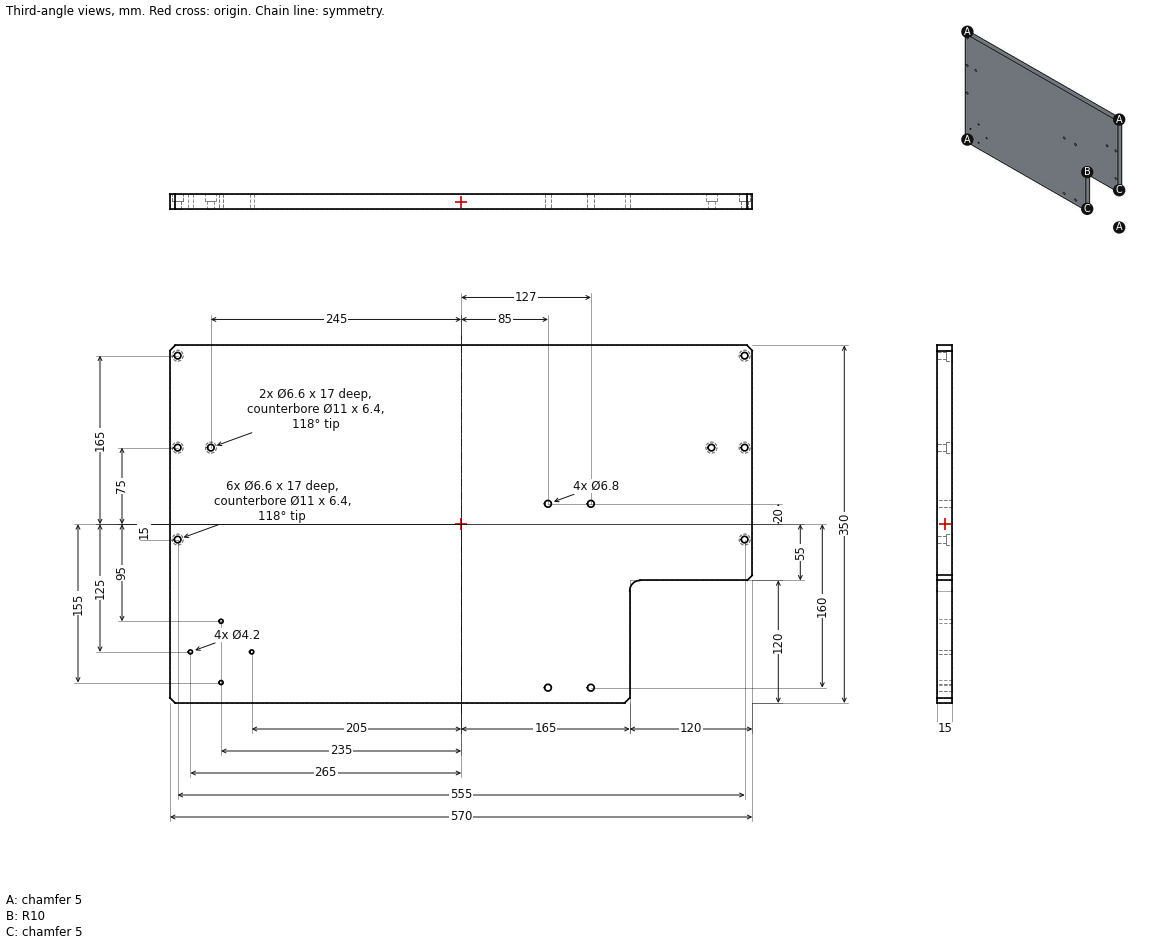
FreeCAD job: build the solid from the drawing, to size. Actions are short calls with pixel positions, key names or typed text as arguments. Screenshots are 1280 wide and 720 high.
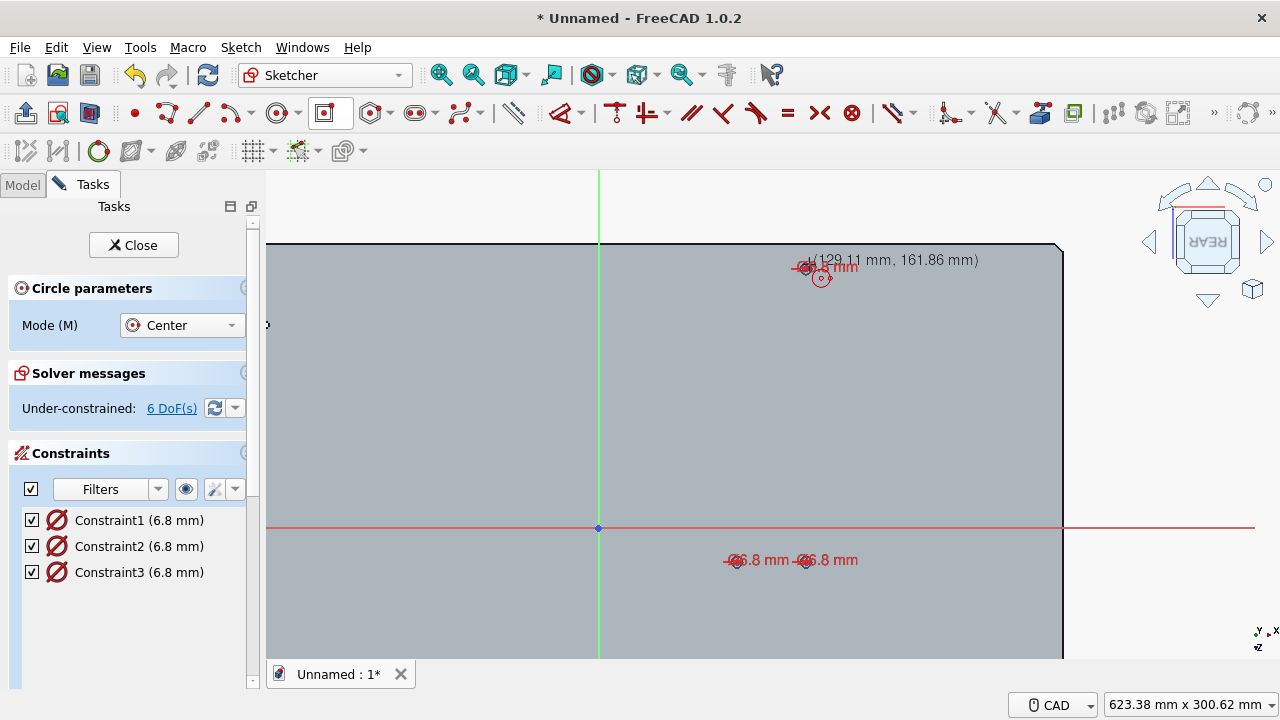
scroll(737, 268, up, 8)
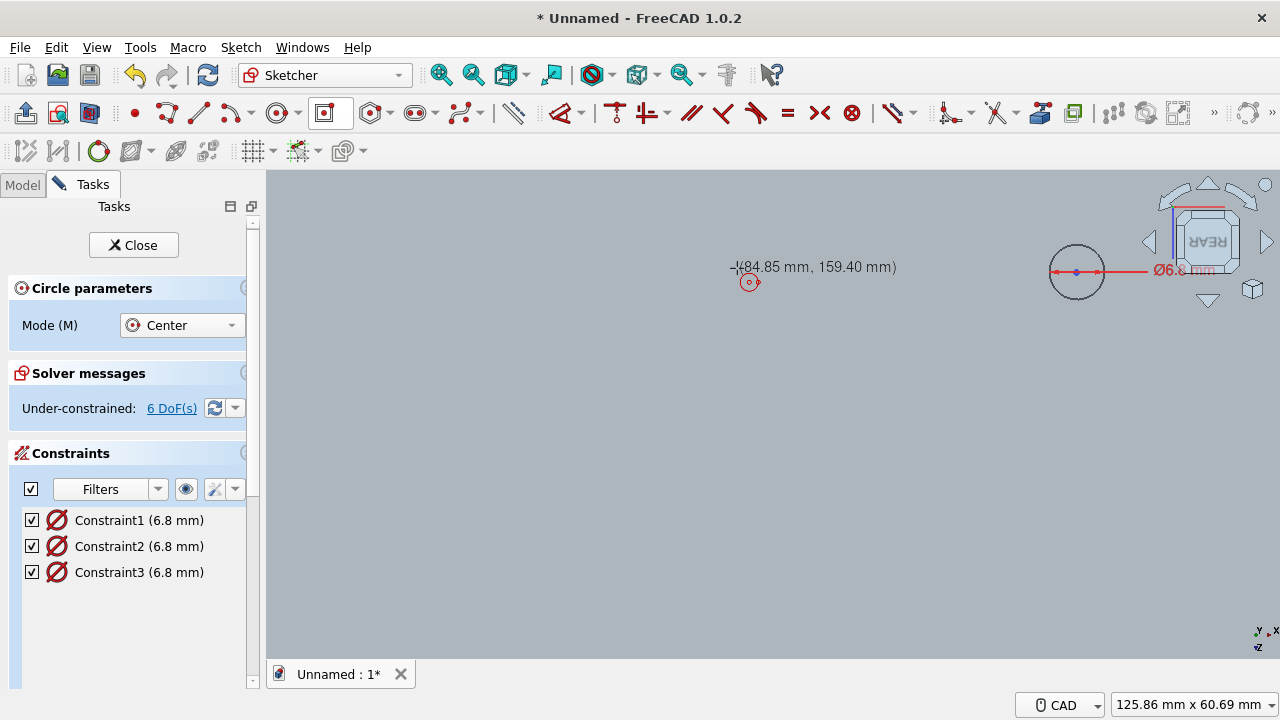
scroll(737, 268, down, 8)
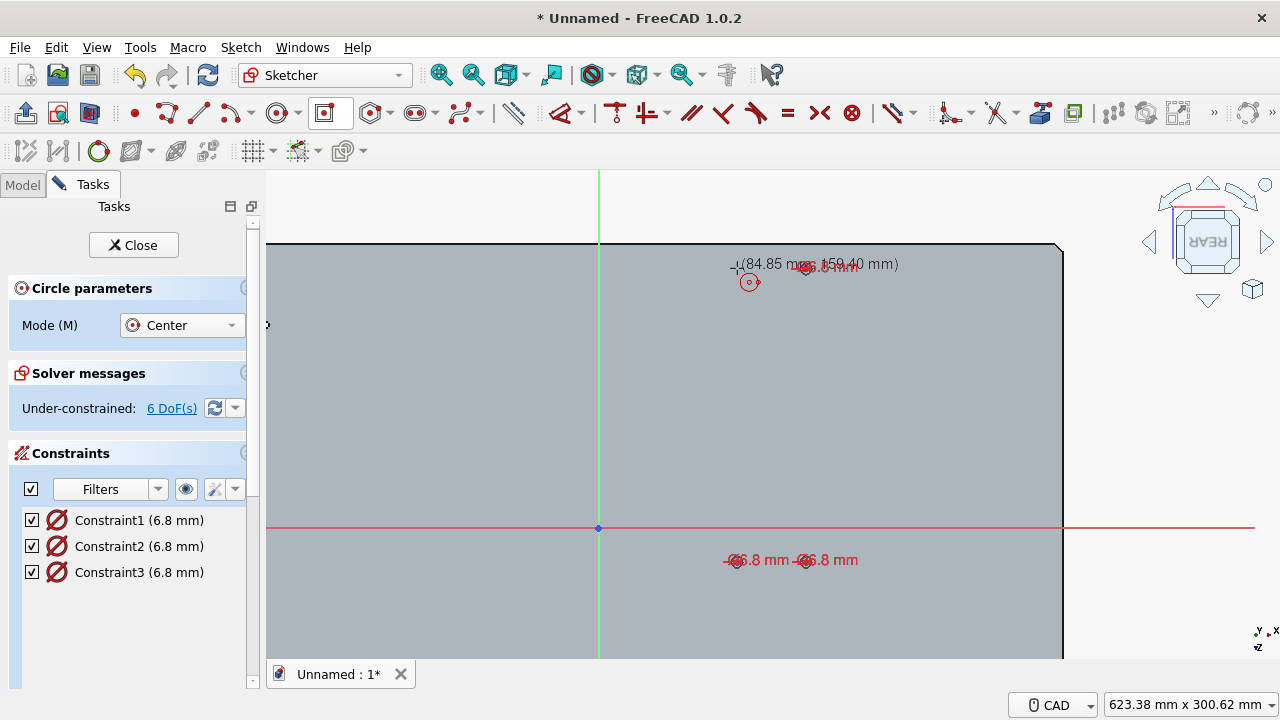
click(737, 268)
move(741, 264)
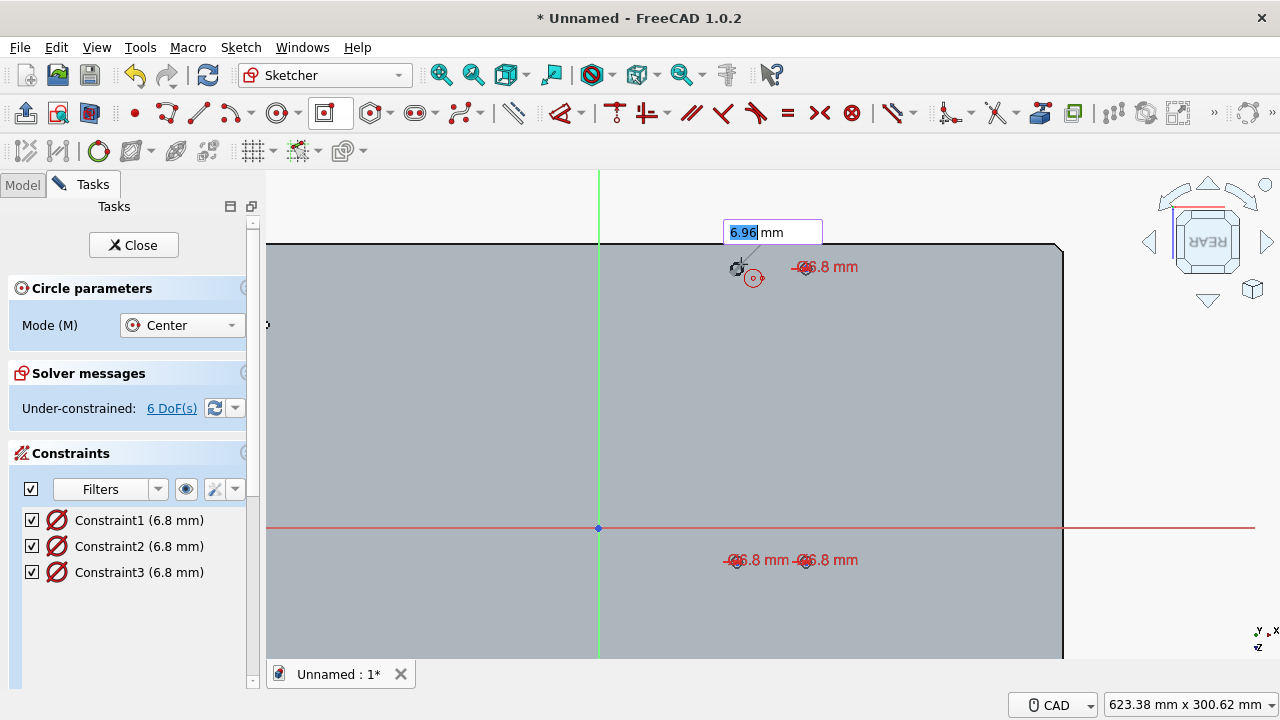
text(6.8)
key(Return)
key(Escape)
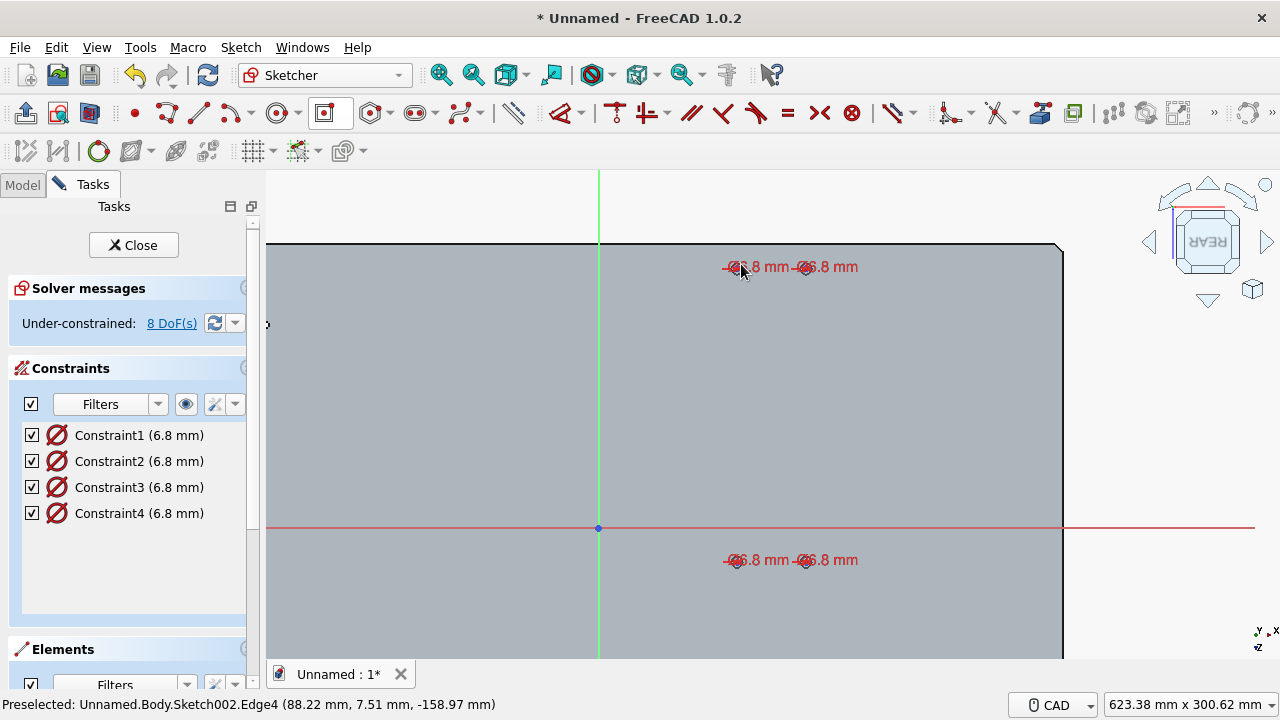
click(560, 114)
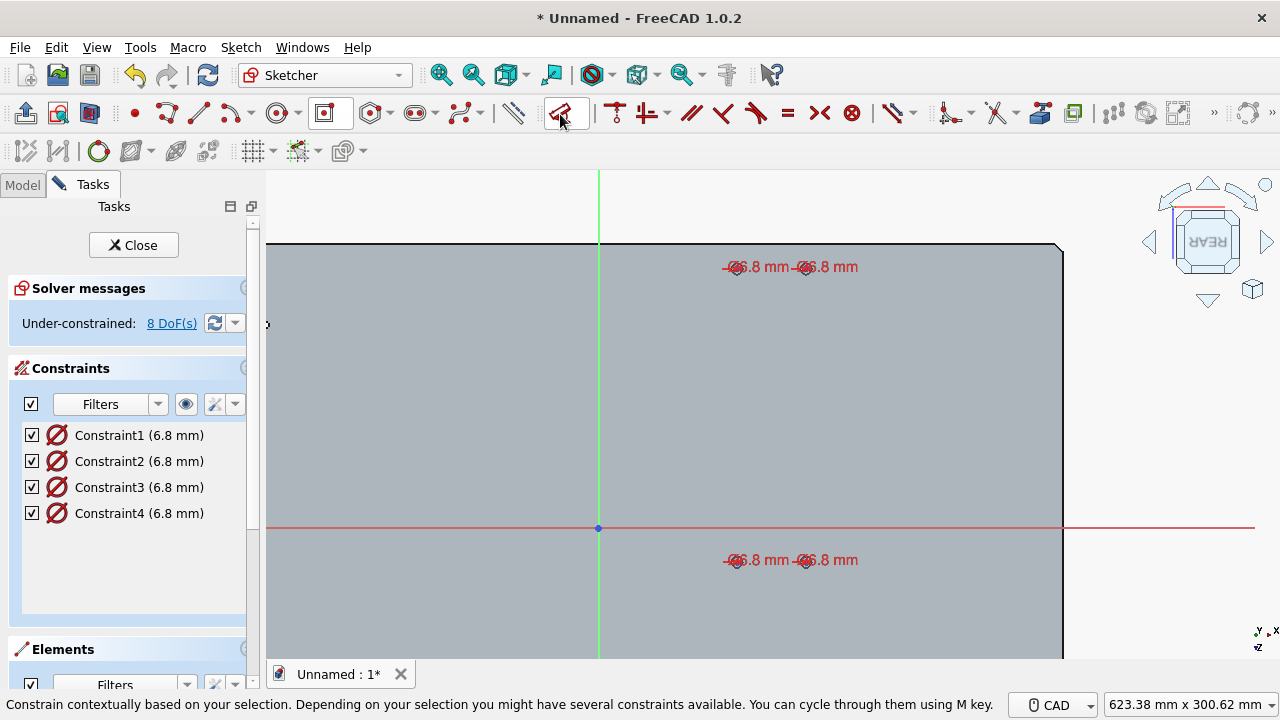
click(737, 562)
click(668, 596)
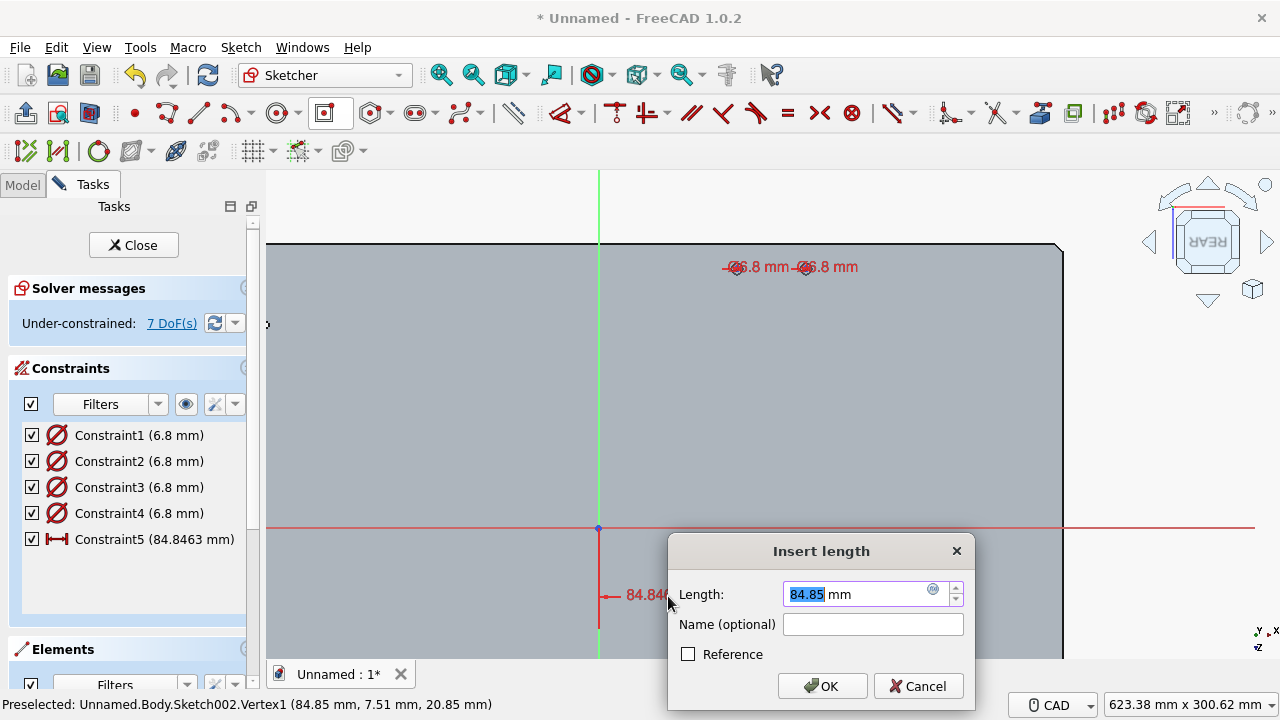
text(85)
key(Return)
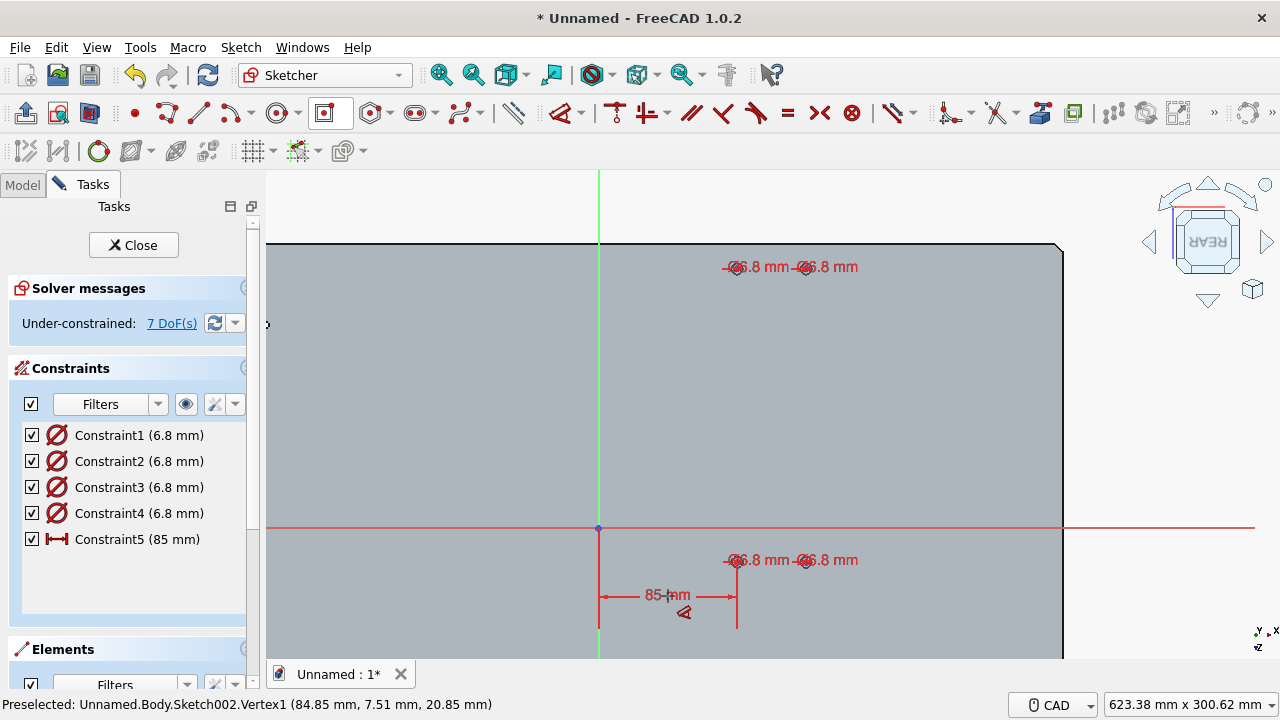
click(737, 562)
click(565, 545)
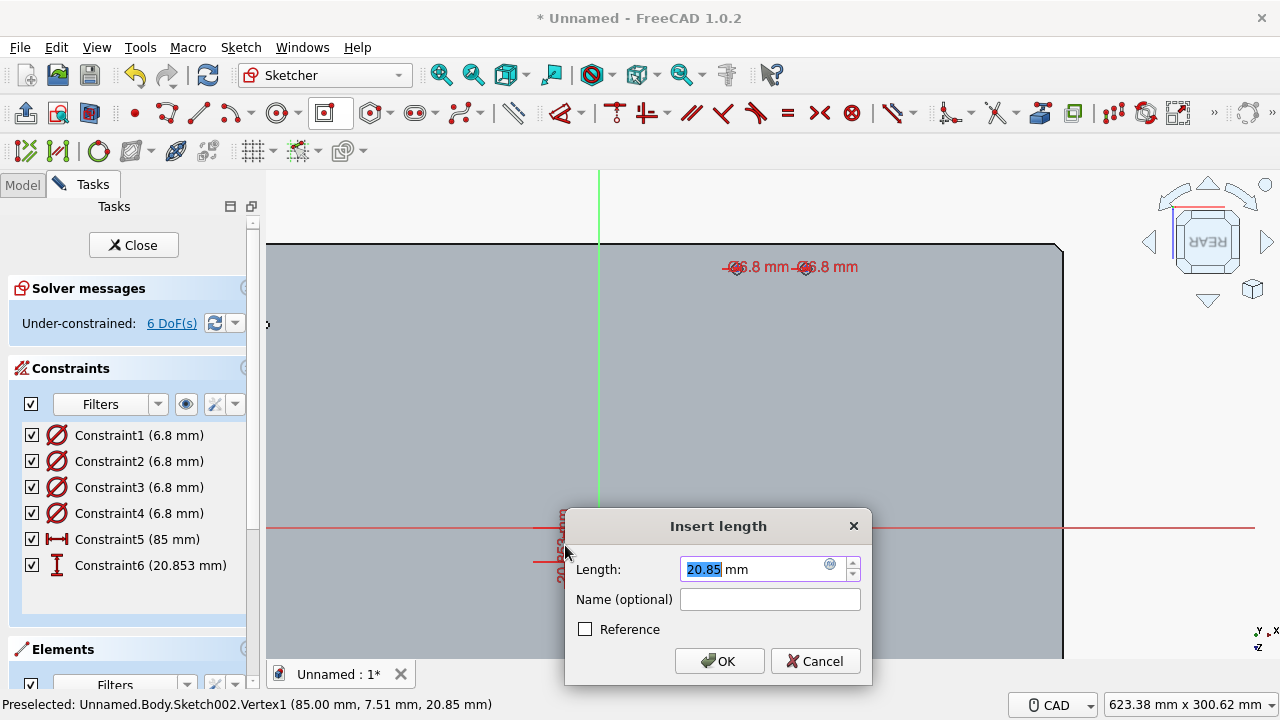
text(20)
key(Return)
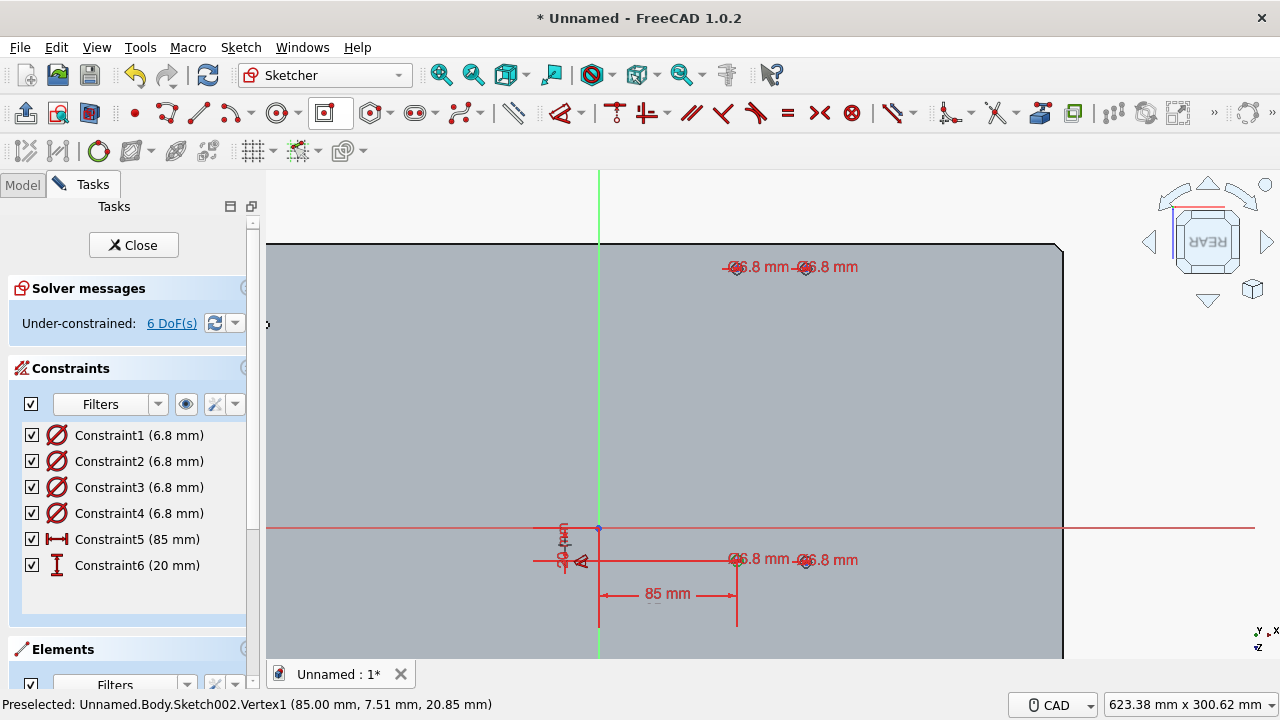
click(806, 562)
click(840, 545)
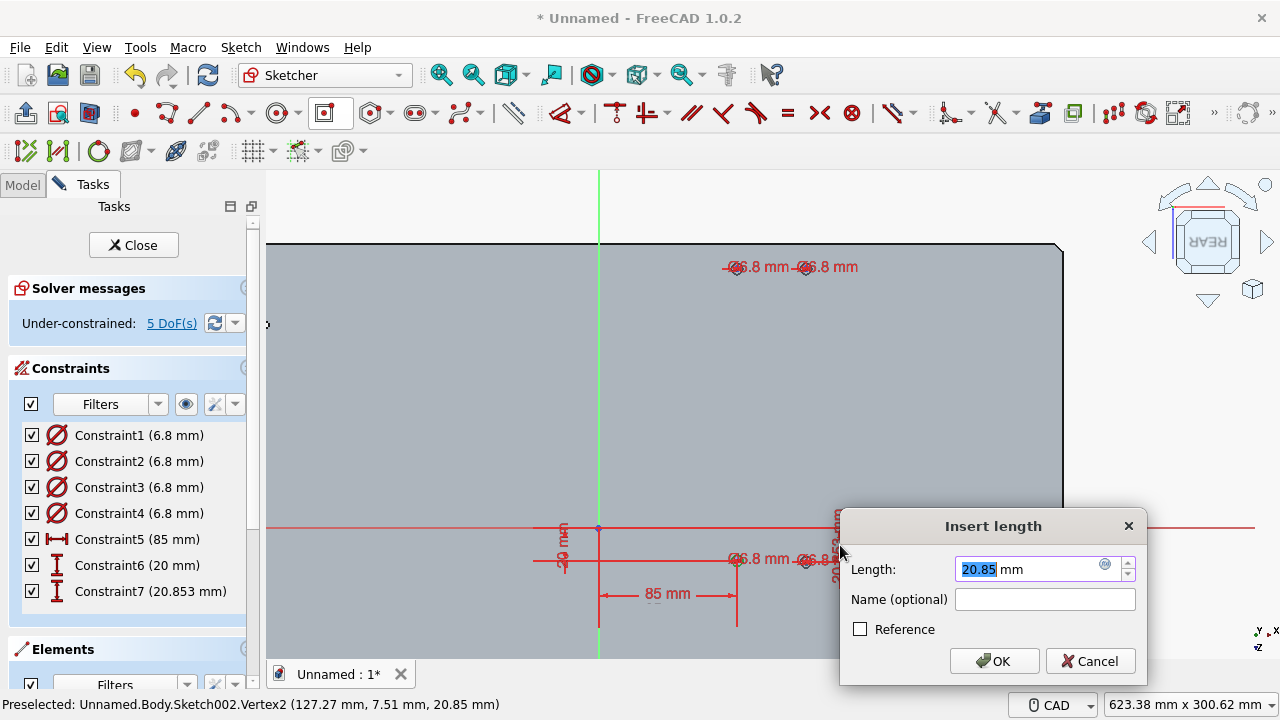
text(20)
key(Return)